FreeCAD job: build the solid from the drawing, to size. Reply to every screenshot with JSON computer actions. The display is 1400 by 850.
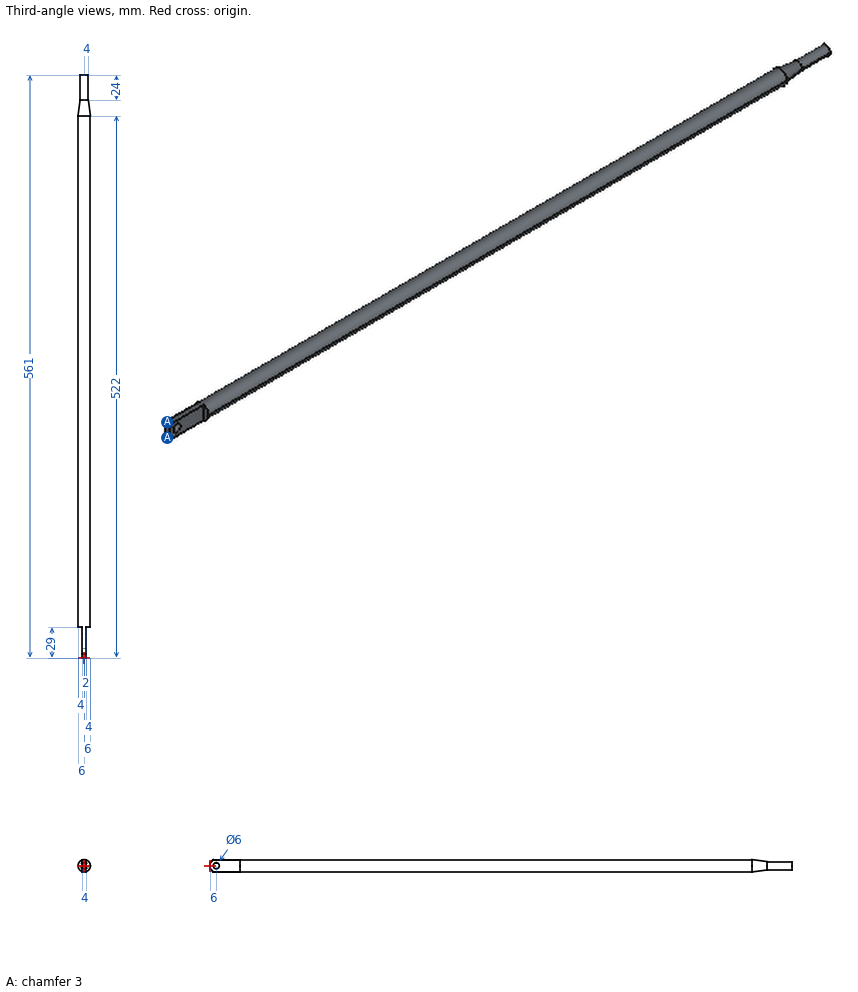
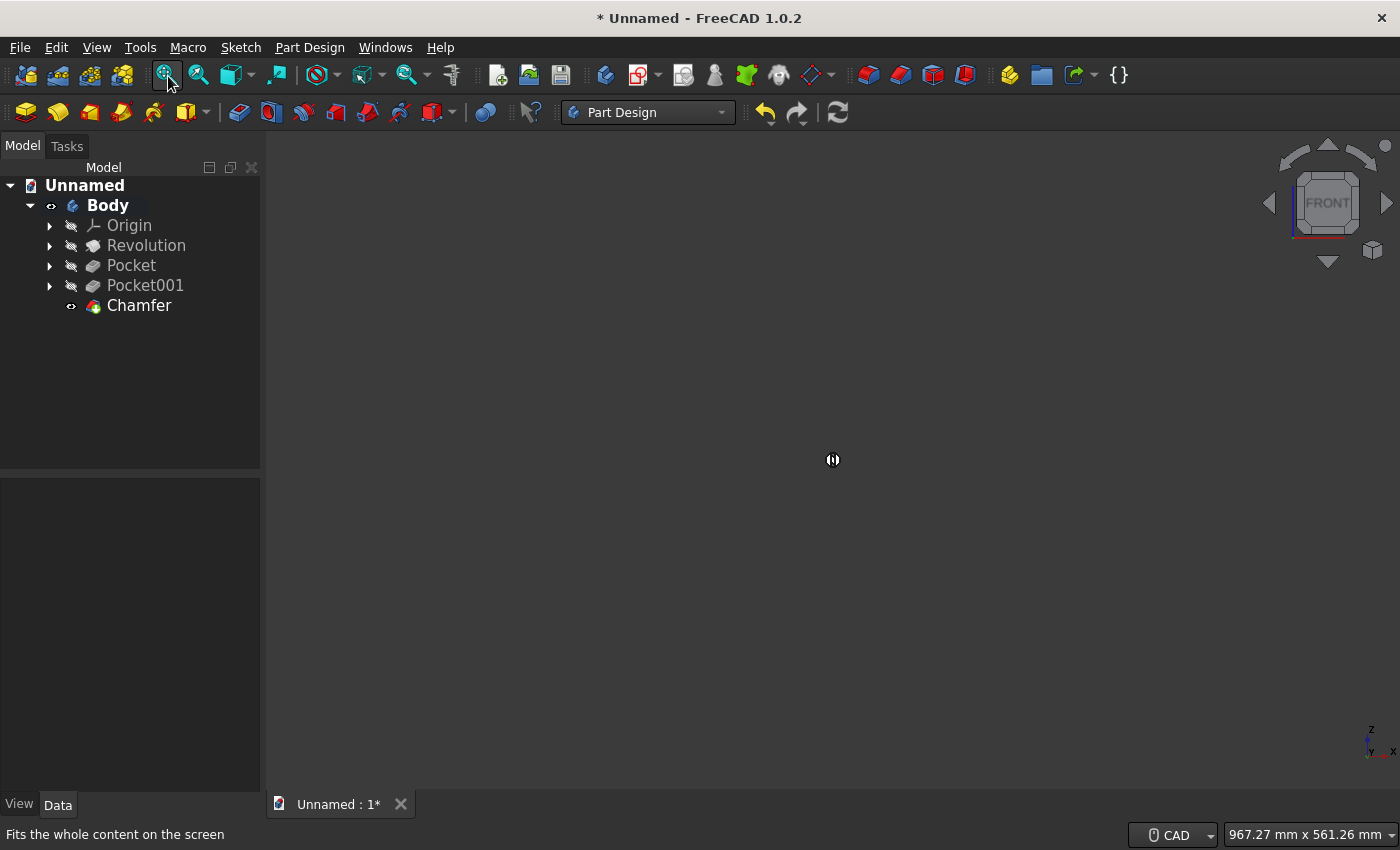
{"action": "key", "text": "6"}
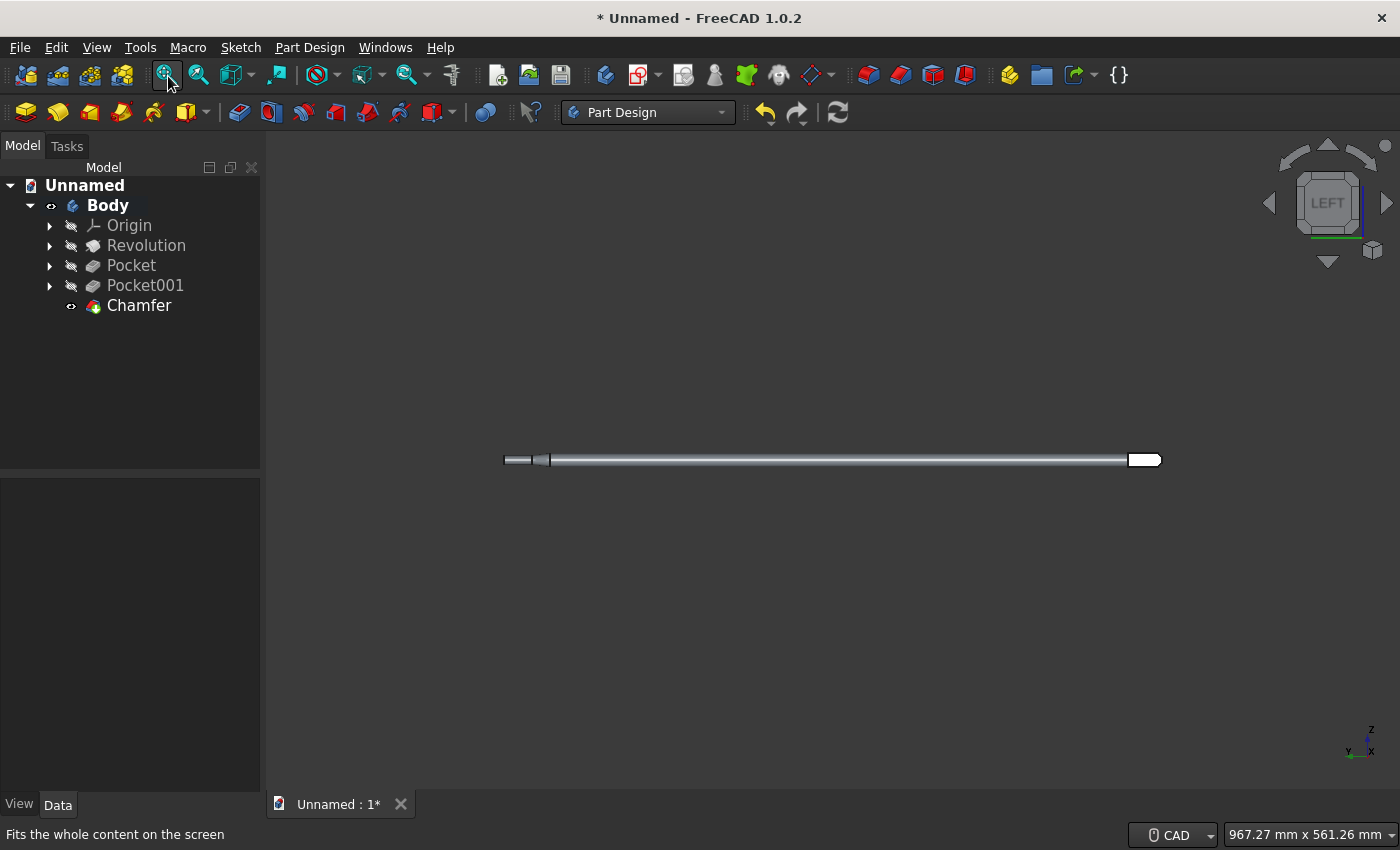
{"action": "scroll", "coordinate": [1135, 459], "scroll_direction": "up", "scroll_amount": 3}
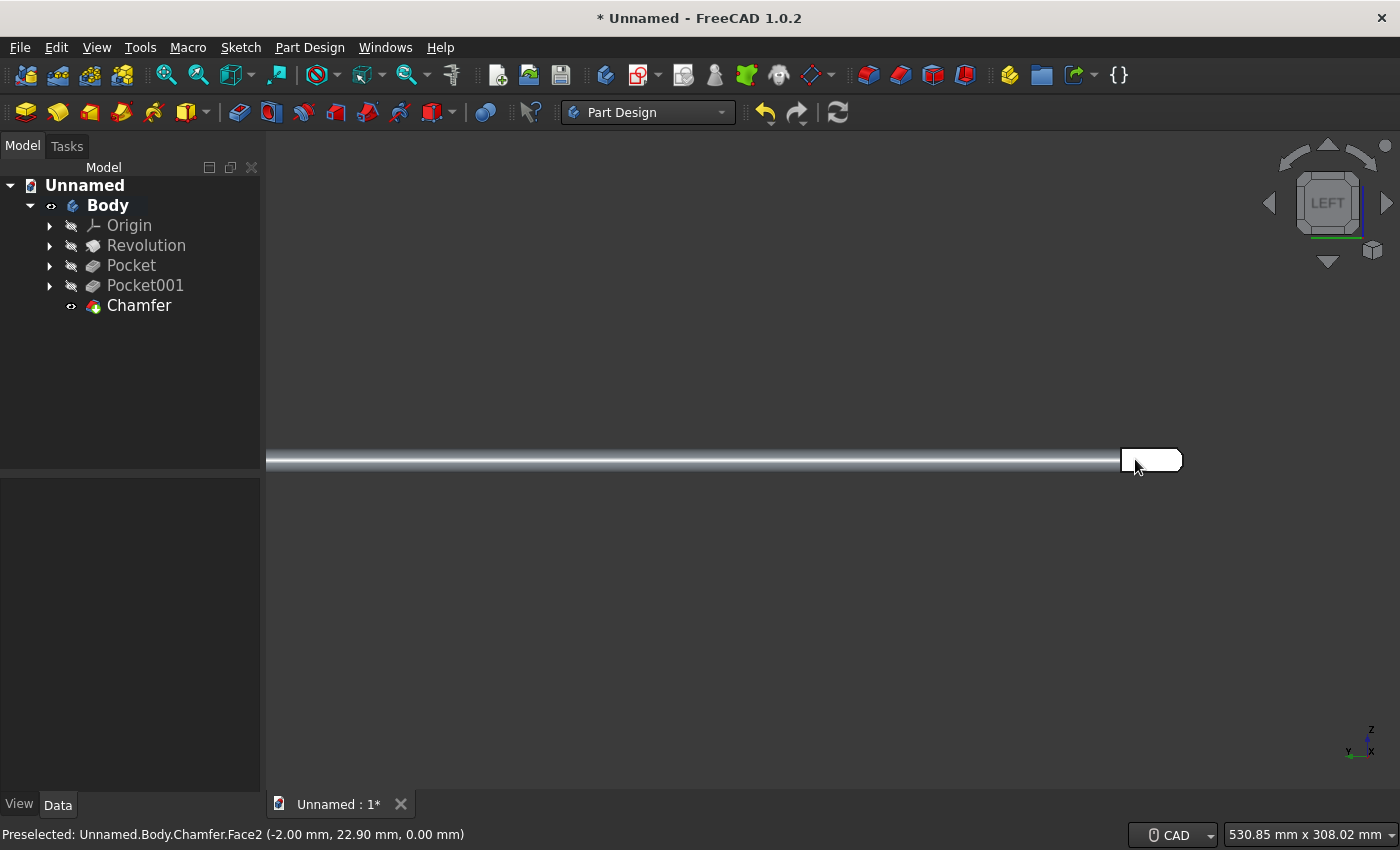
{"action": "left_click", "coordinate": [1135, 459]}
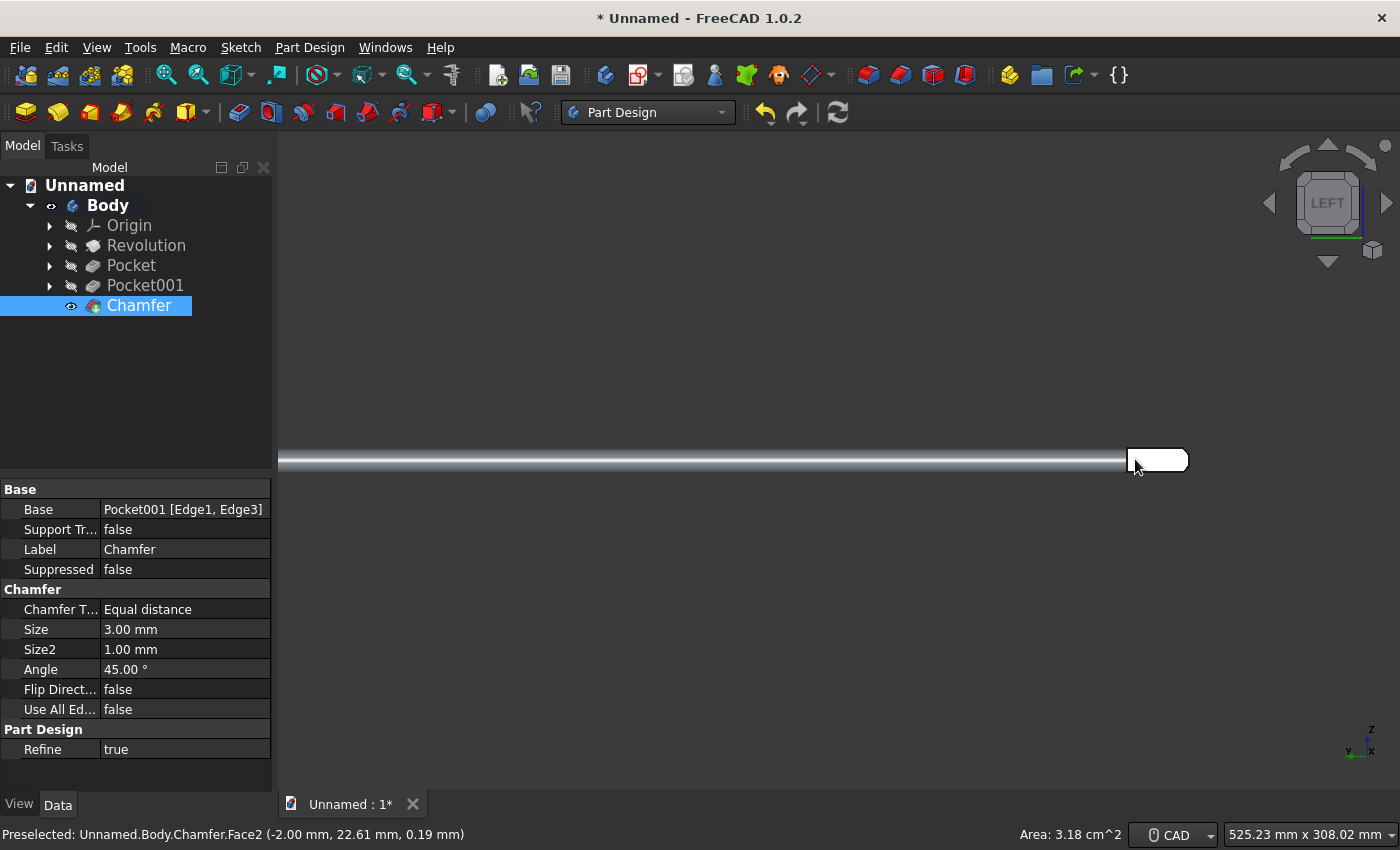
{"action": "left_click", "coordinate": [638, 76]}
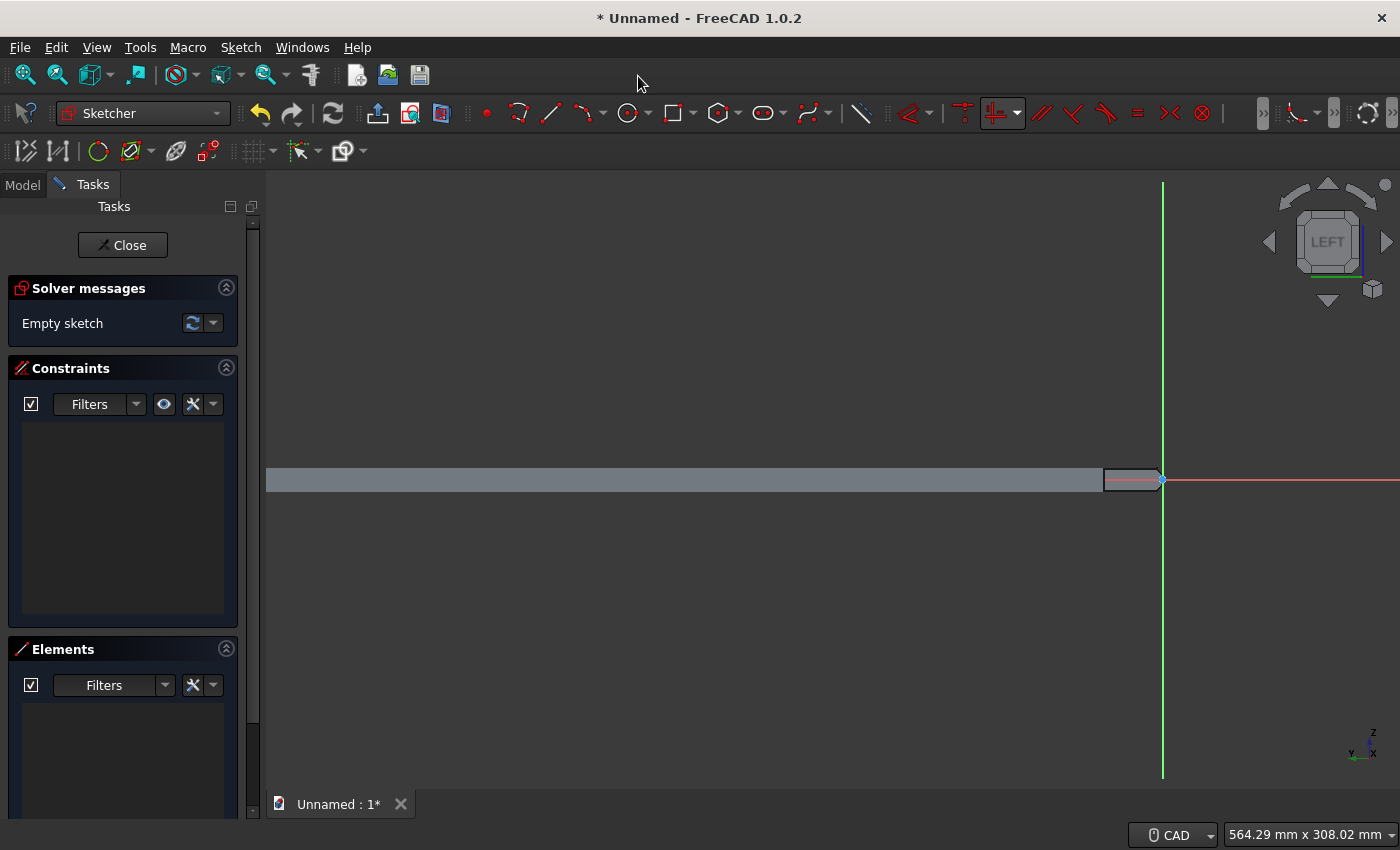
{"action": "left_click", "coordinate": [442, 114]}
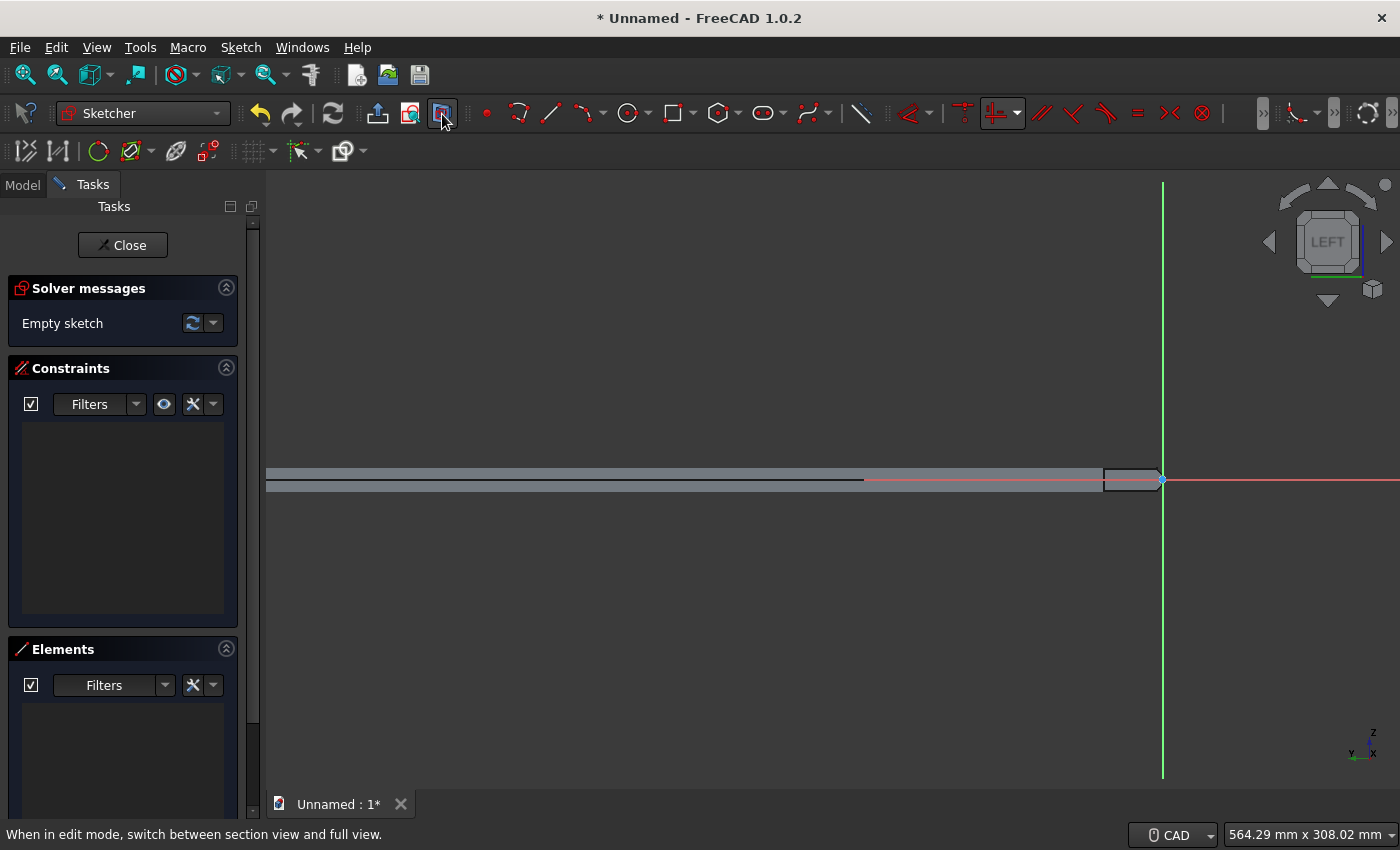
{"action": "scroll", "coordinate": [1174, 480], "scroll_direction": "up", "scroll_amount": 15}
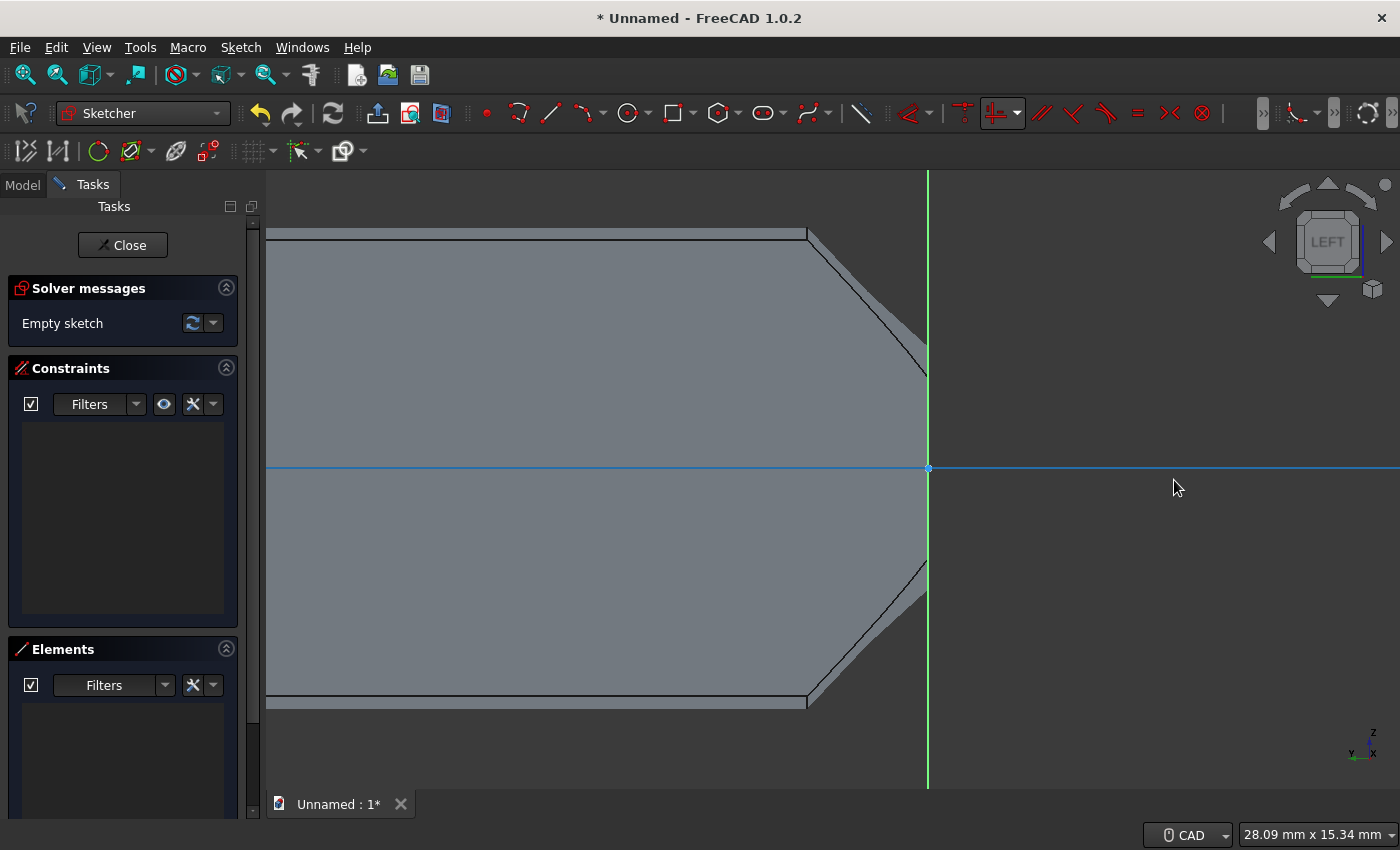
{"action": "scroll", "coordinate": [711, 445], "scroll_direction": "up", "scroll_amount": 2}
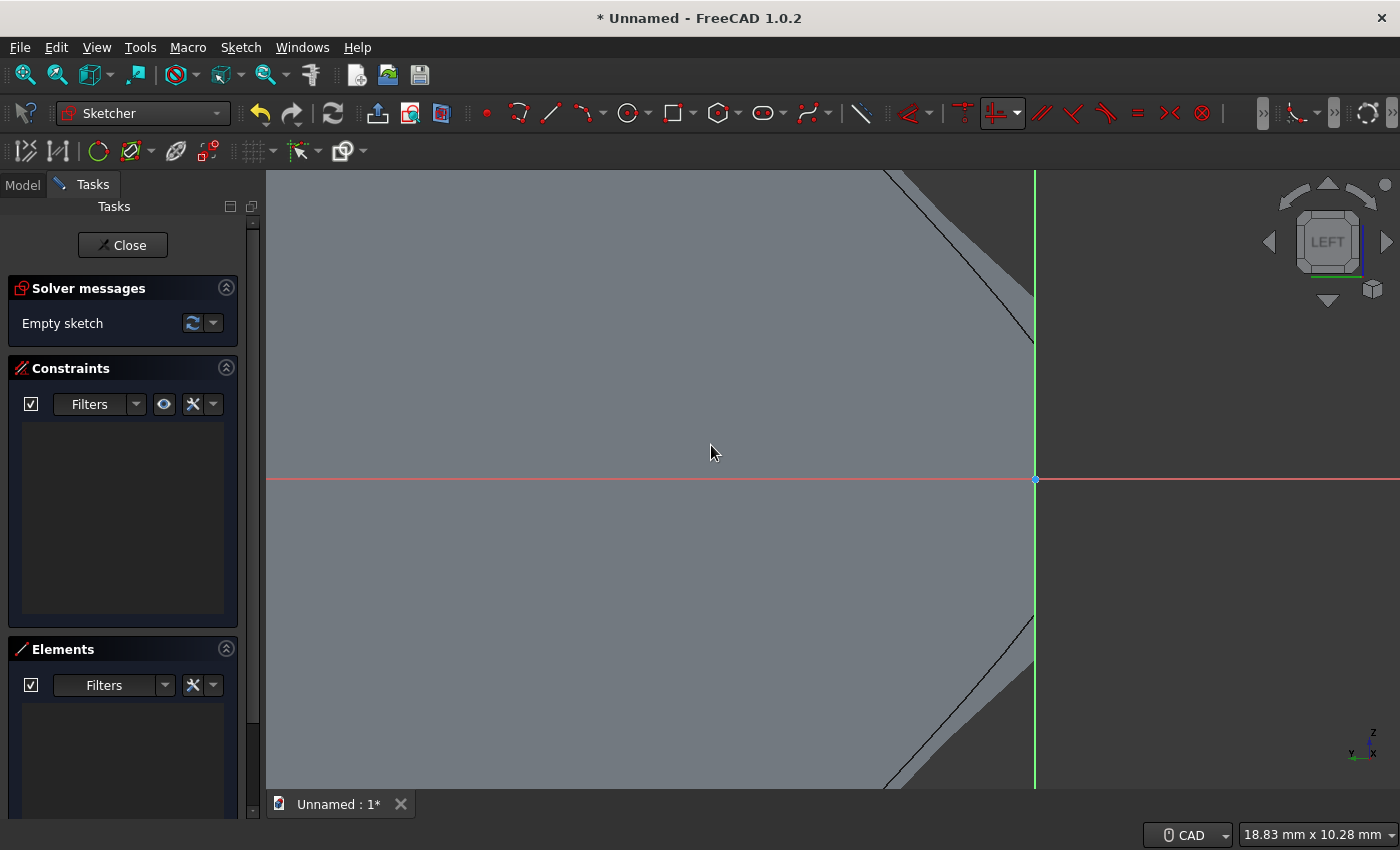
{"action": "left_click", "coordinate": [628, 114]}